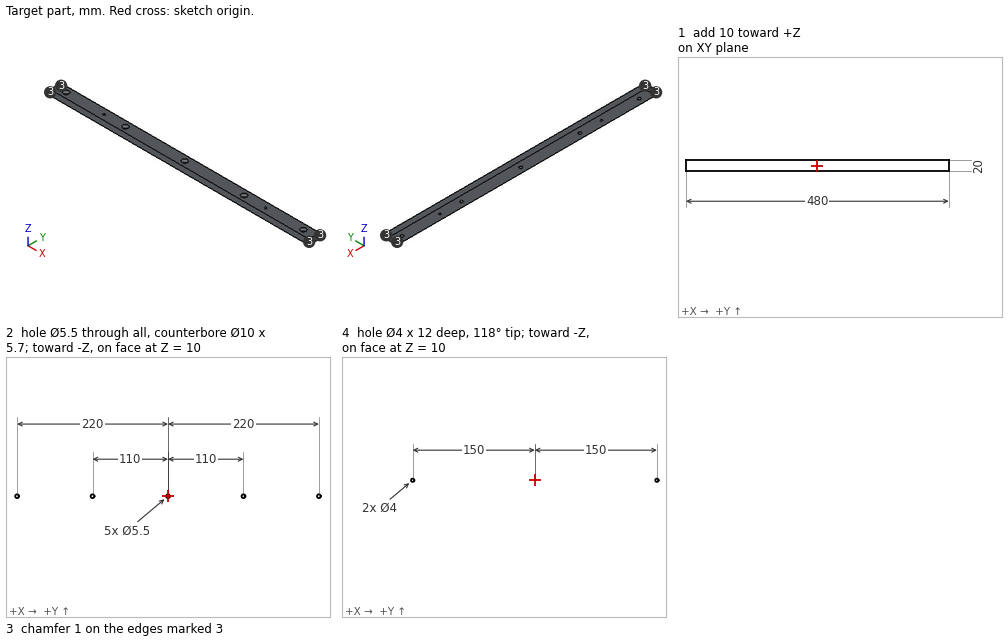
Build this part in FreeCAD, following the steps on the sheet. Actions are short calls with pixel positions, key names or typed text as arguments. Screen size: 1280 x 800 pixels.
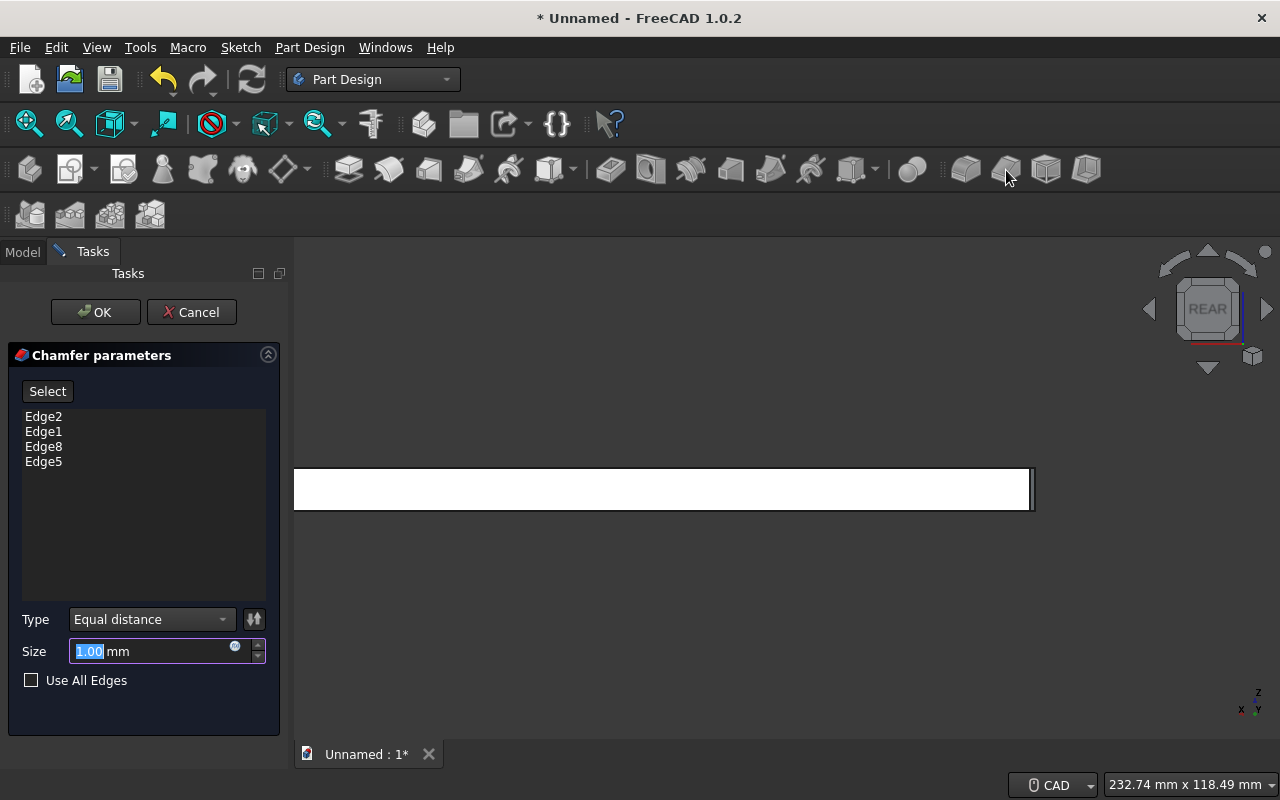
text(1)
key(Tab)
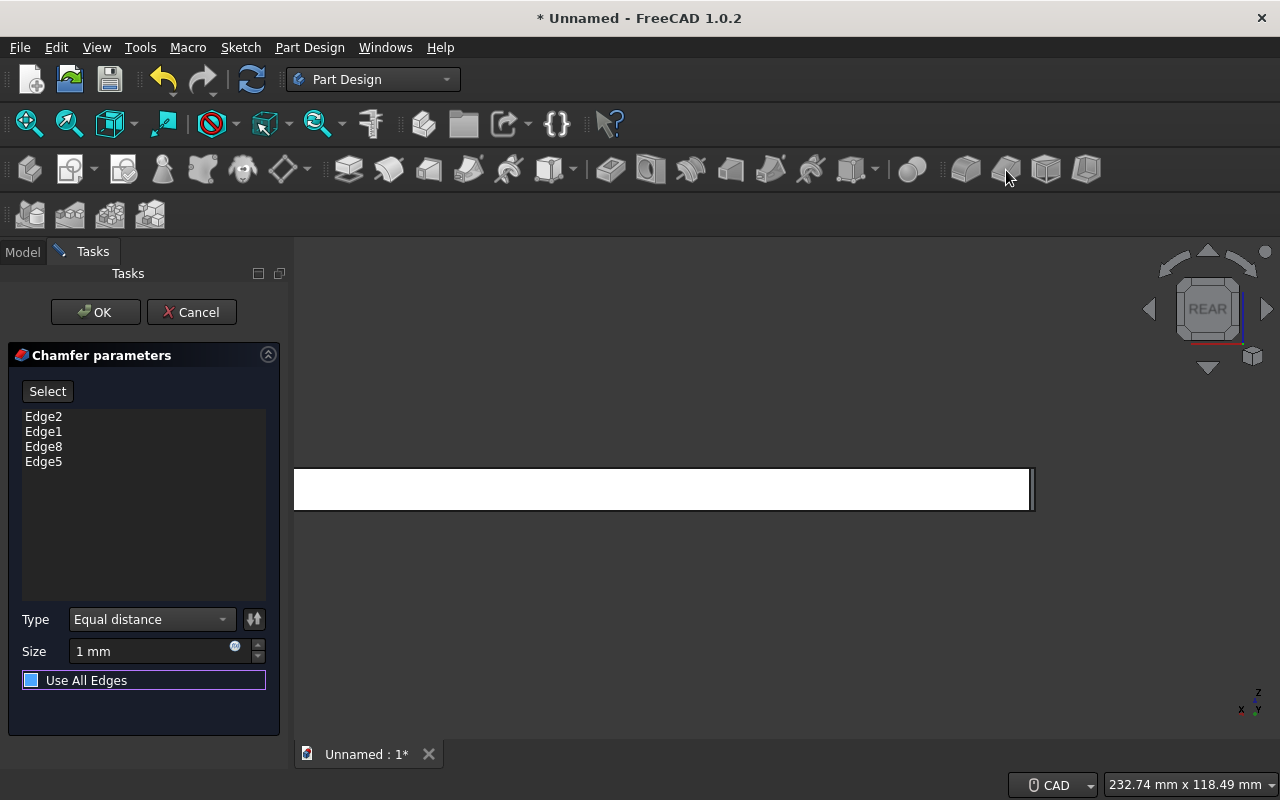
click(96, 312)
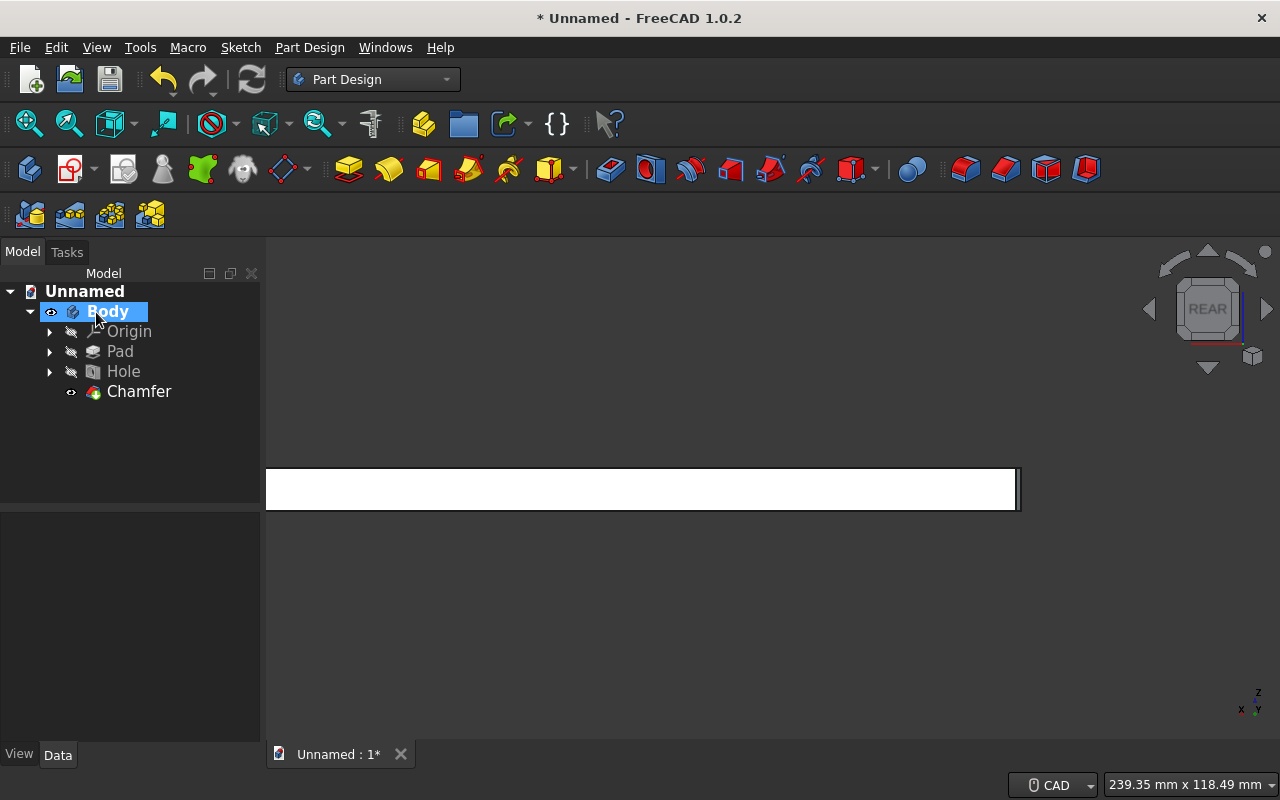
click(30, 124)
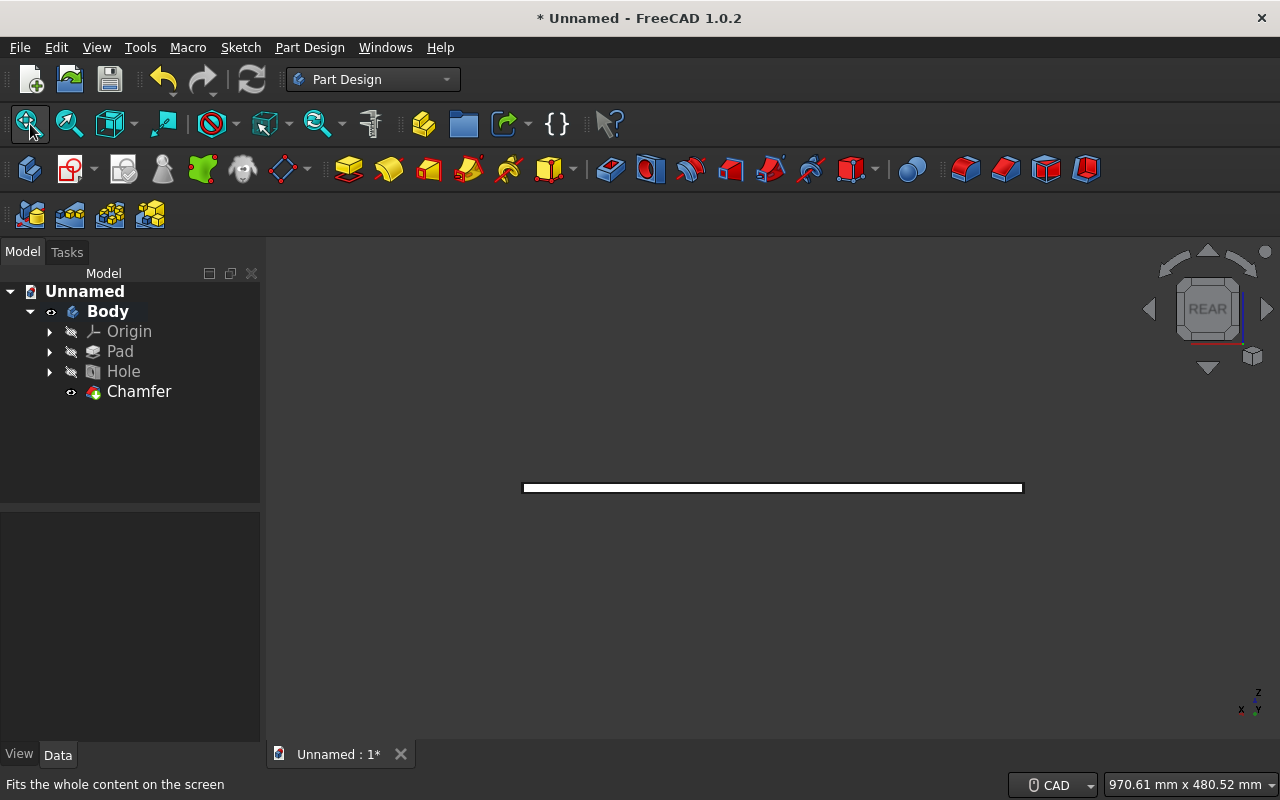
key(0)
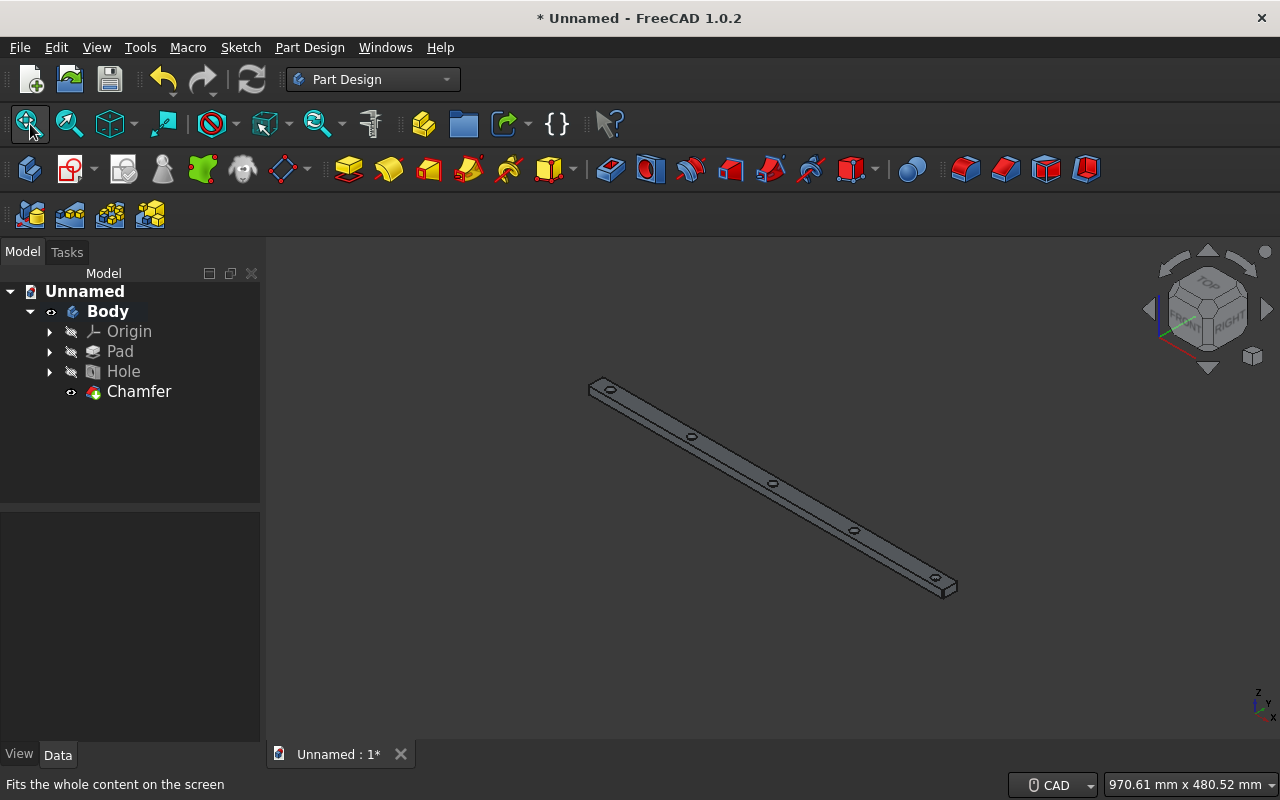
click(30, 124)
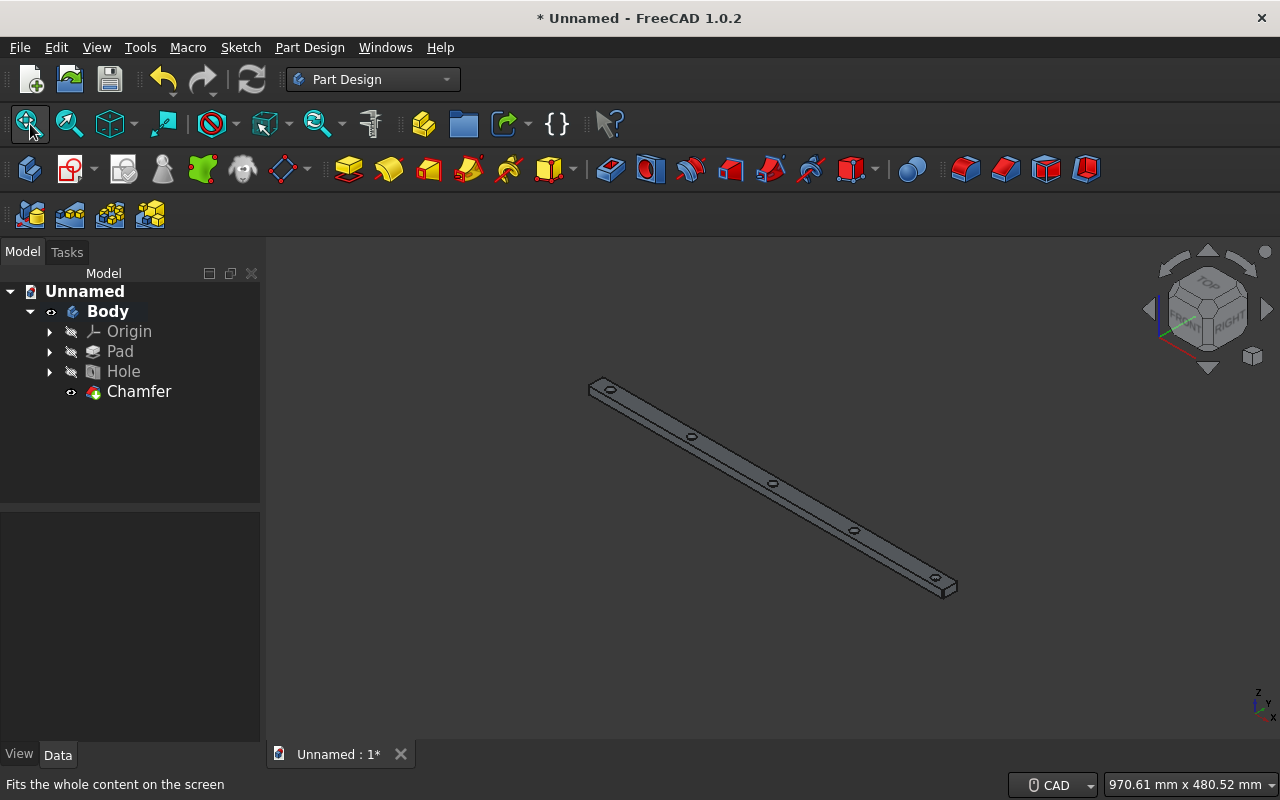
key(2)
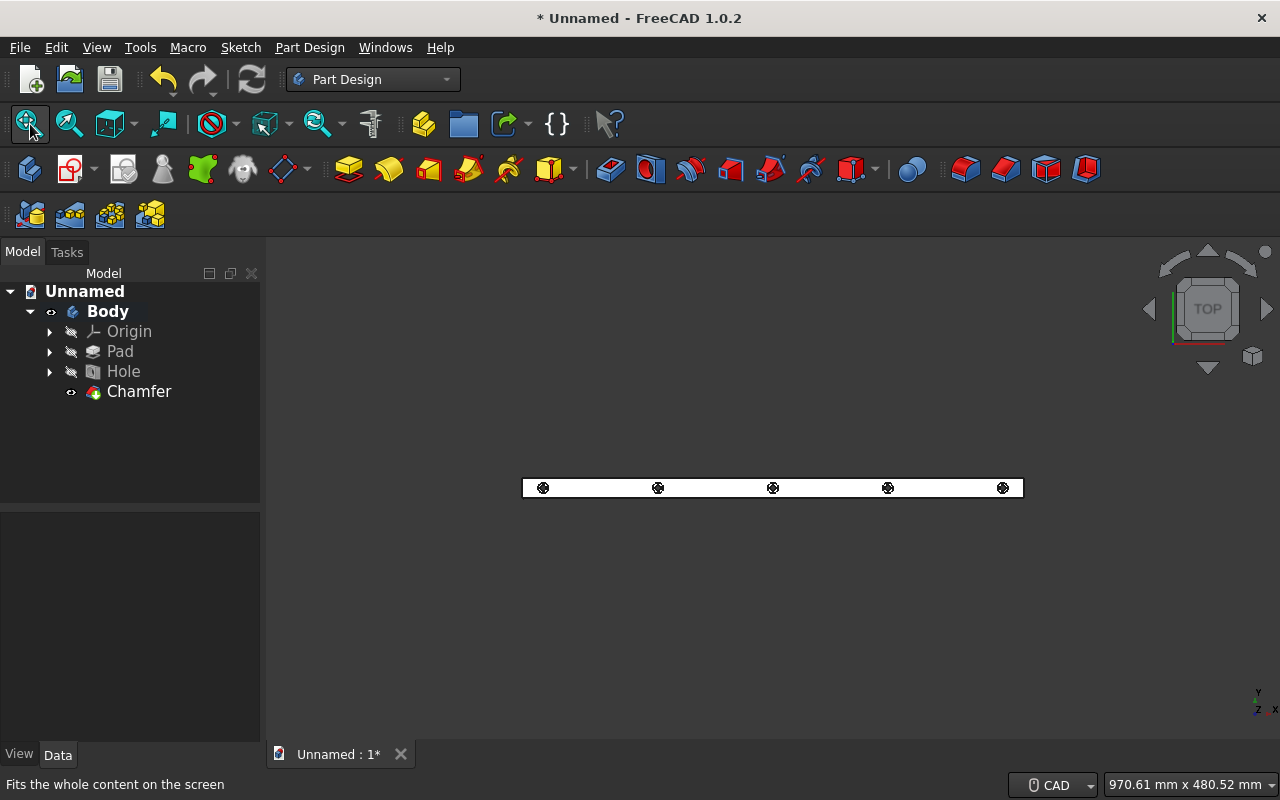
click(916, 487)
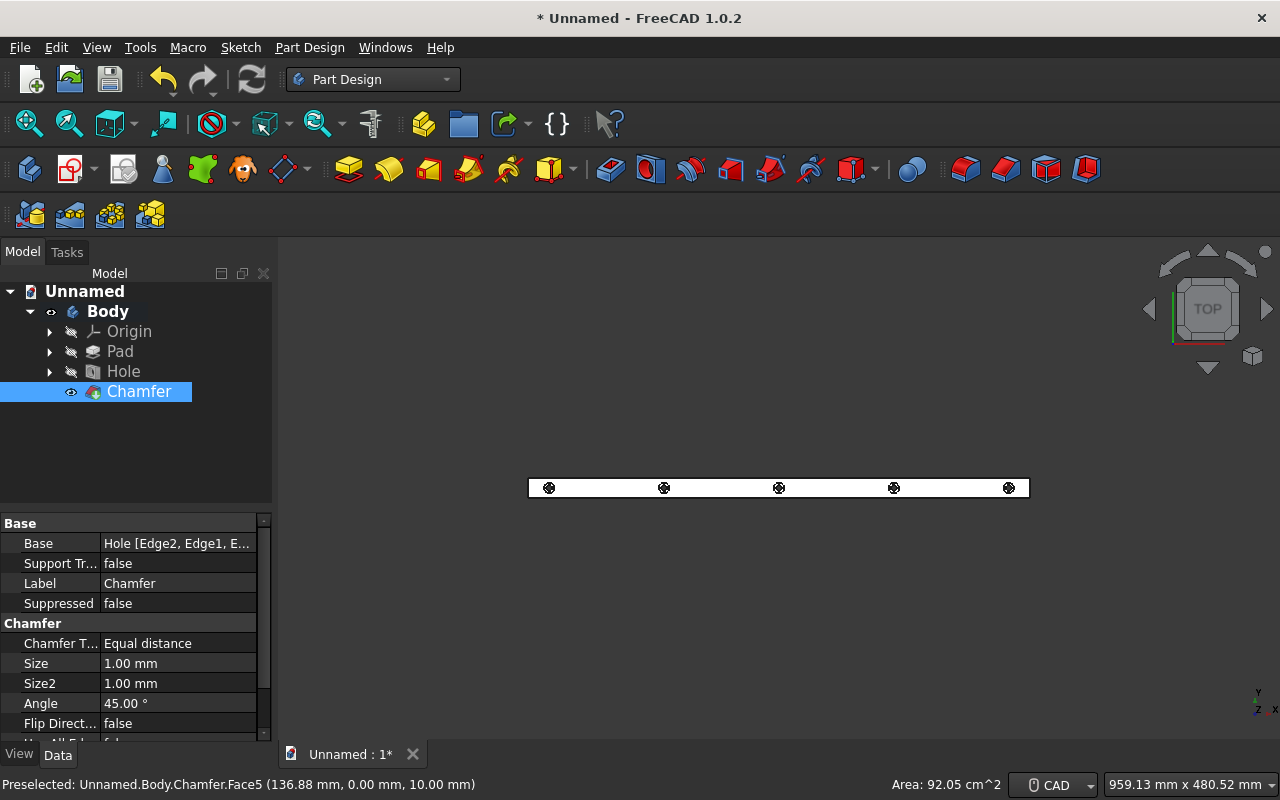
click(70, 170)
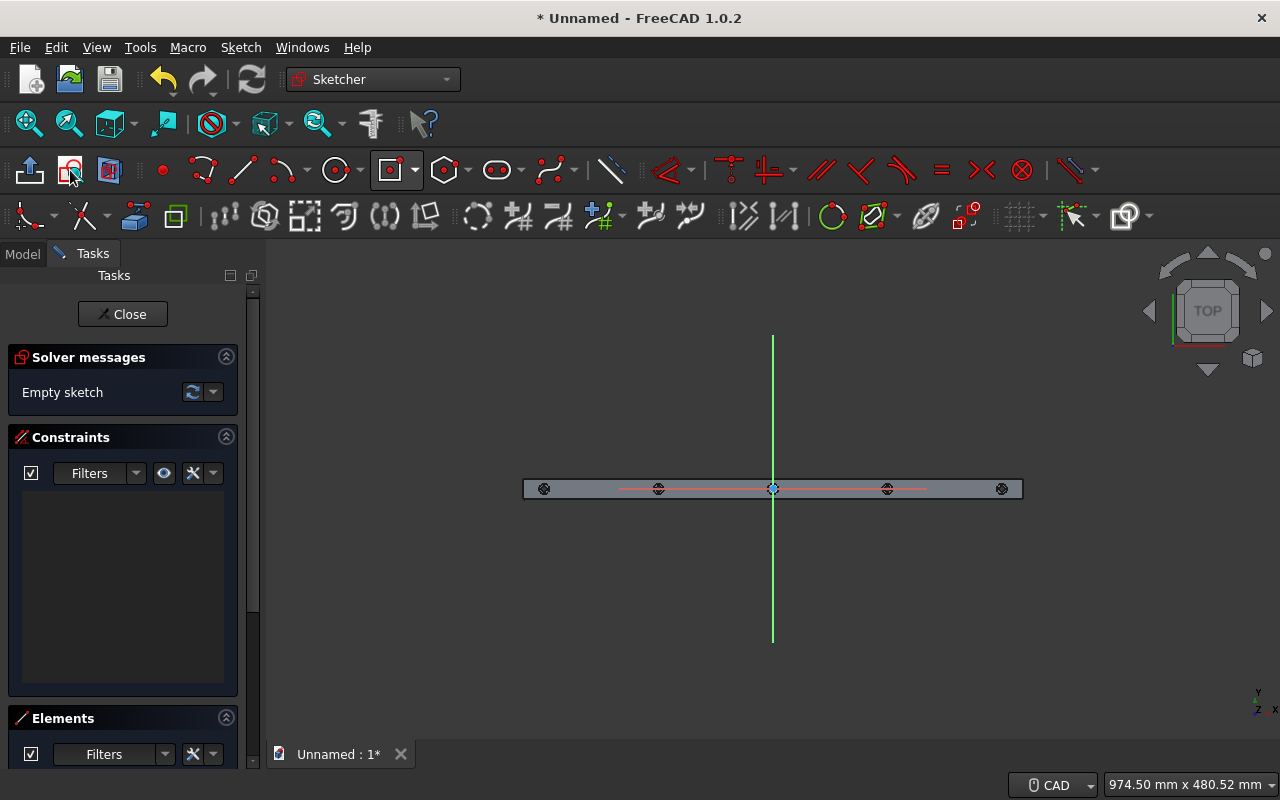
scroll(856, 489, up, 3)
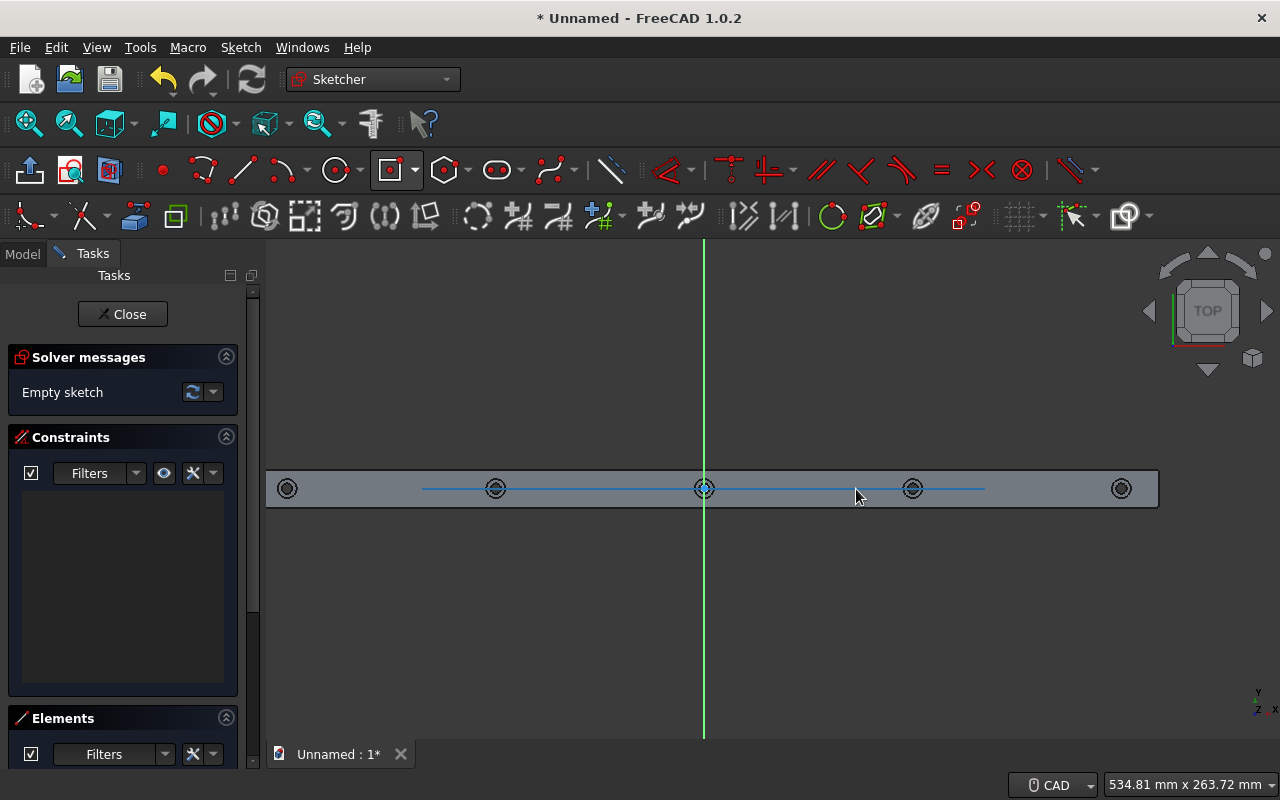
click(336, 170)